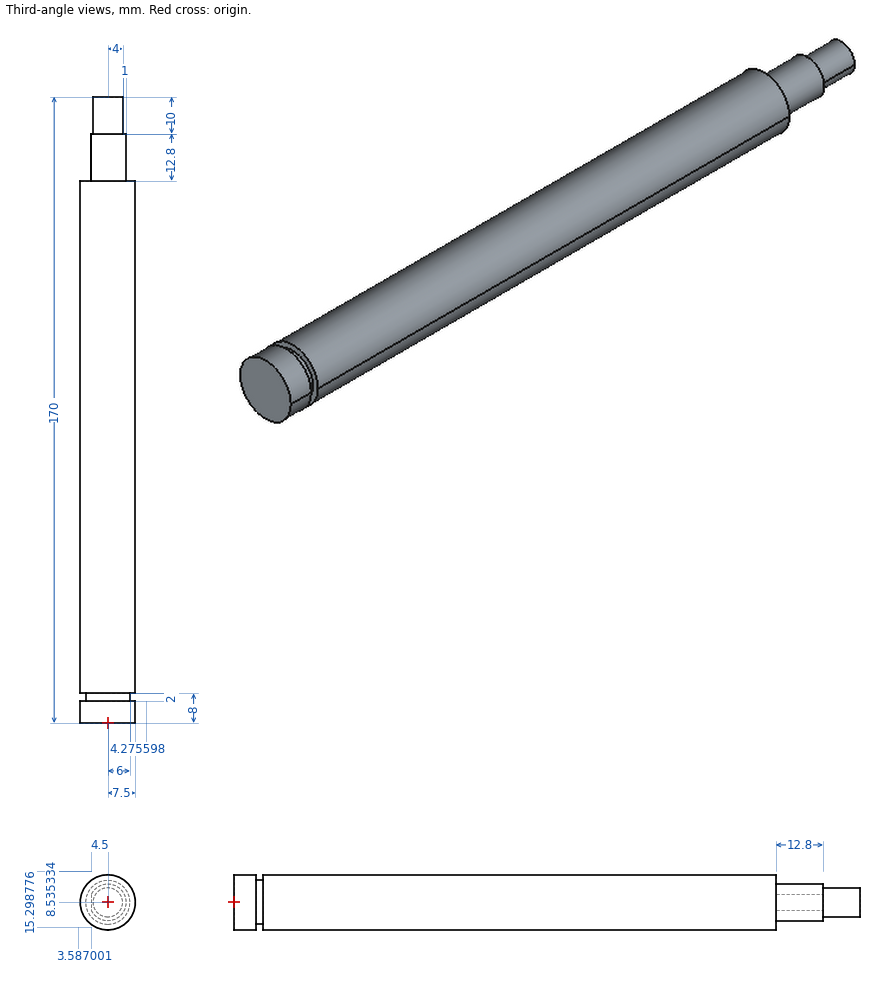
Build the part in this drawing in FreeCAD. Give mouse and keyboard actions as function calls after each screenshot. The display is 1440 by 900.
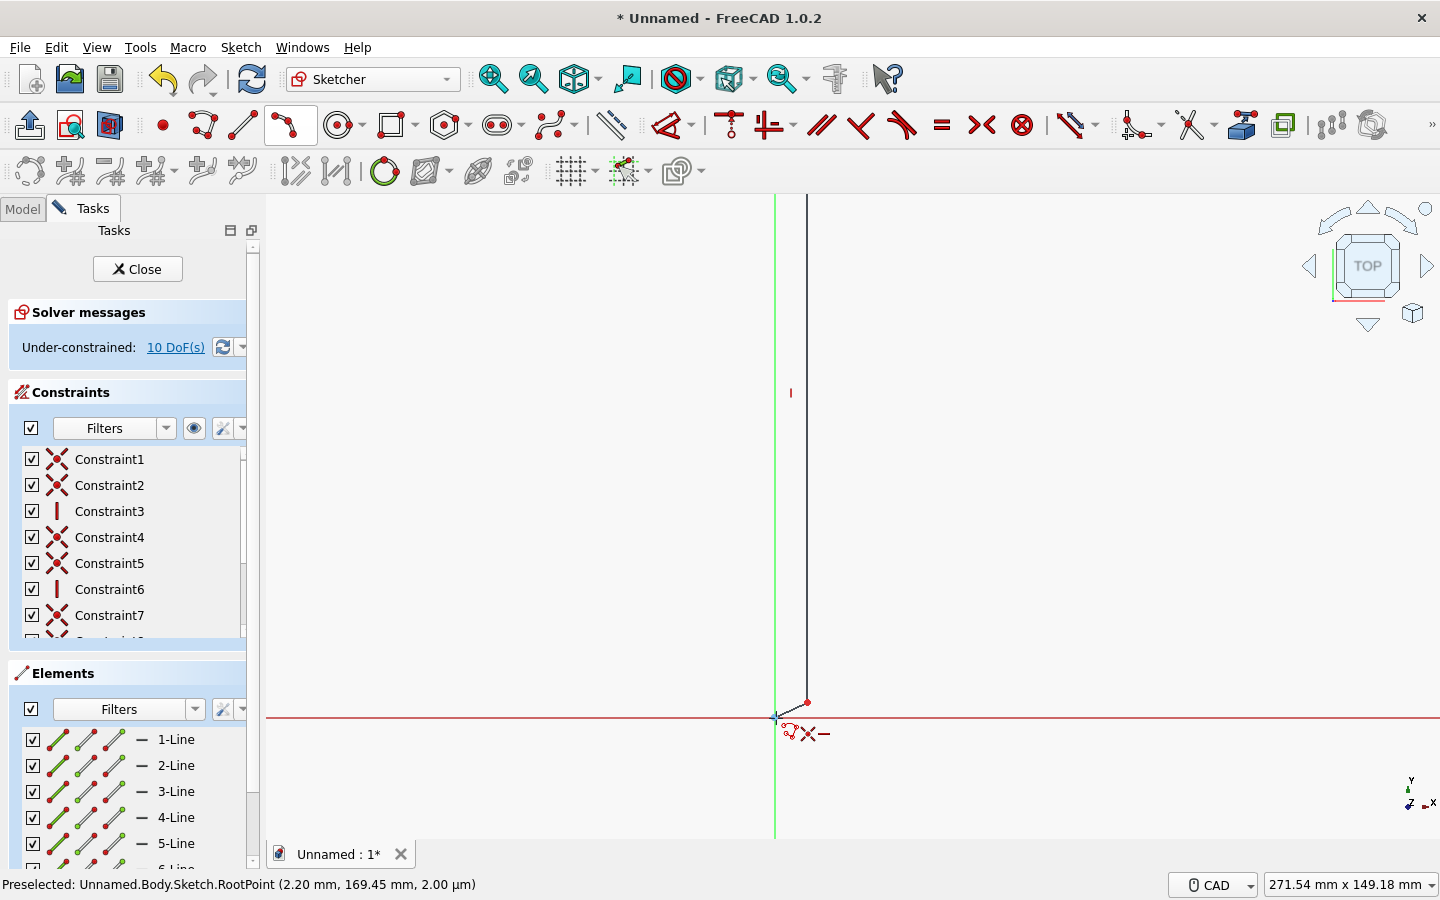
click(775, 718)
key(Escape)
key(Escape)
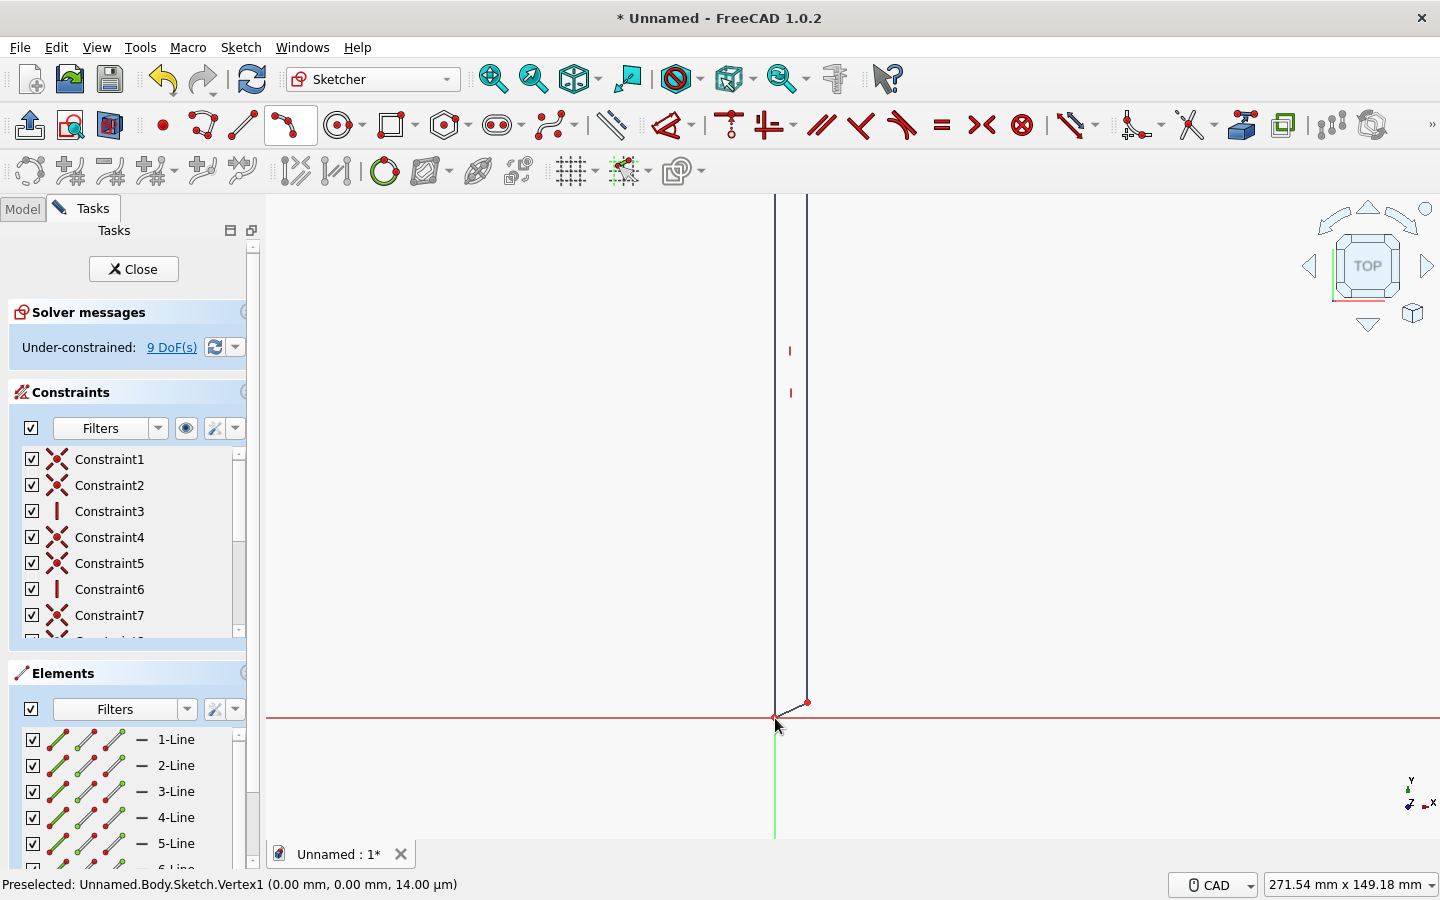
scroll(798, 707, up, 2)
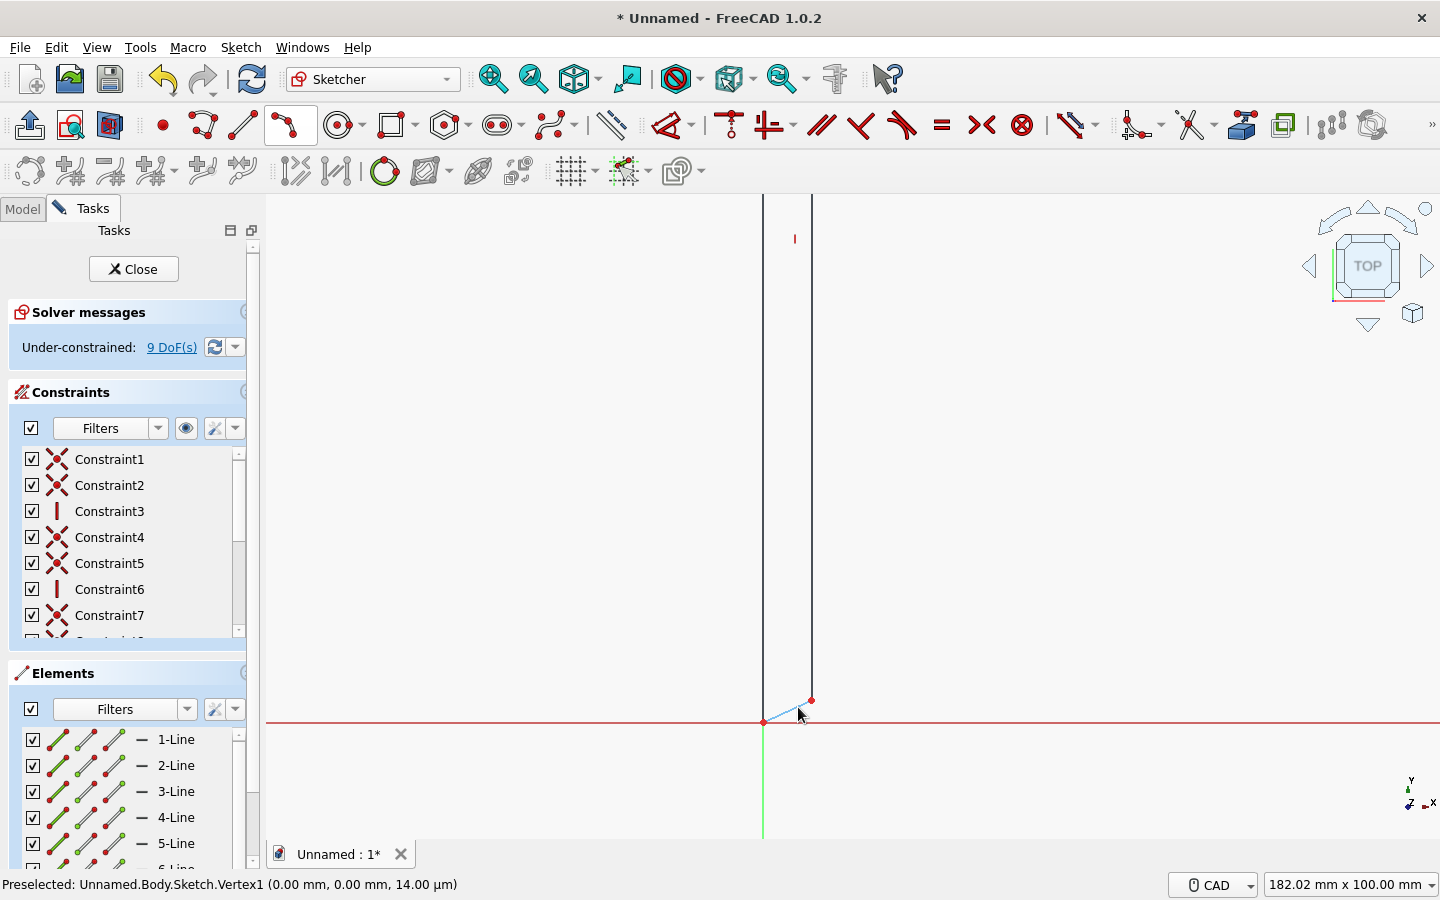
click(797, 707)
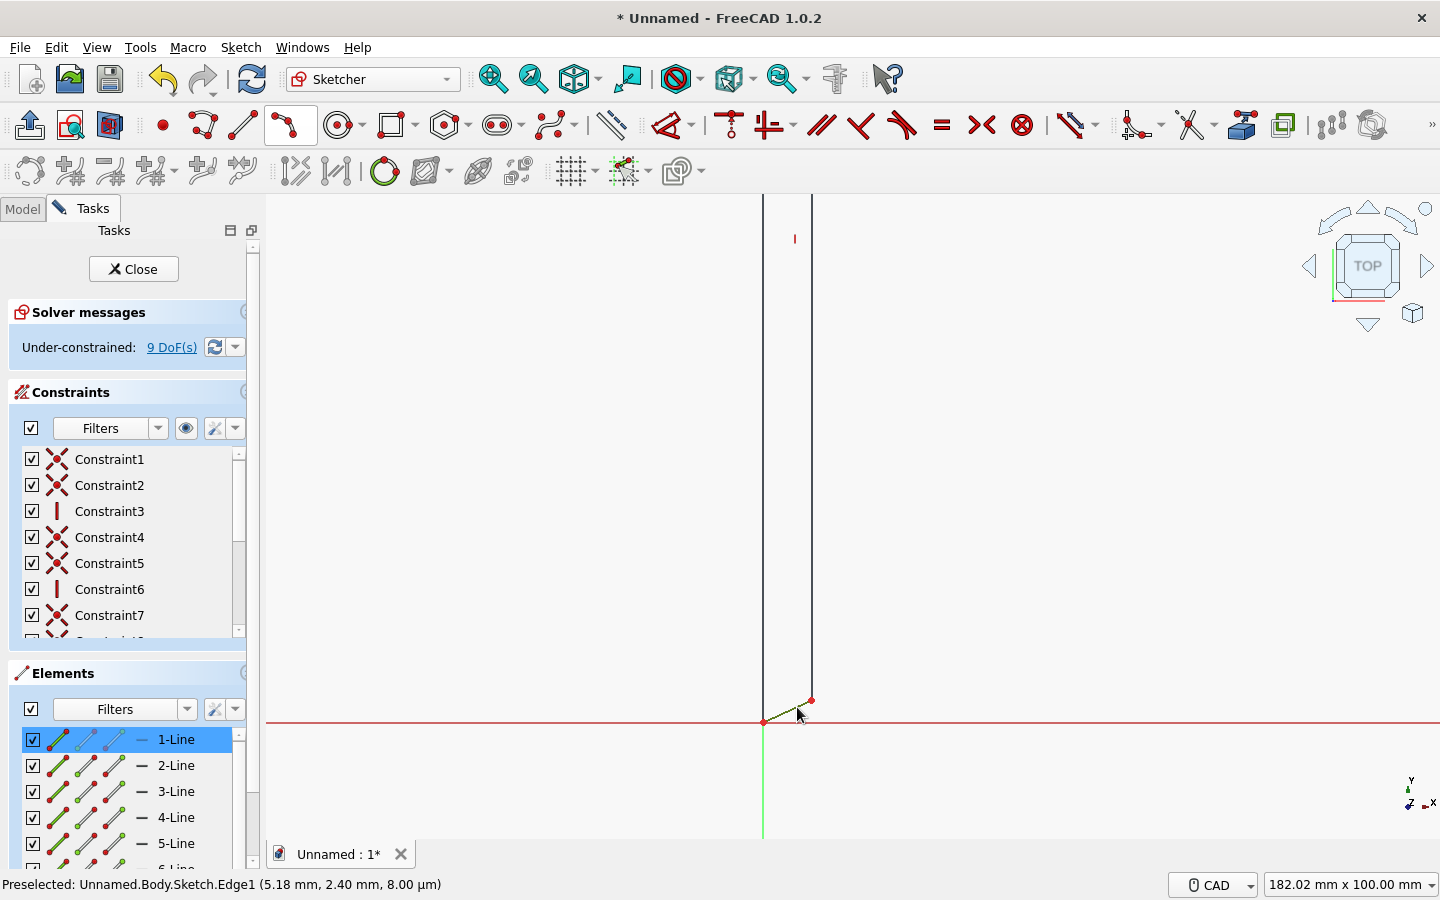
click(796, 126)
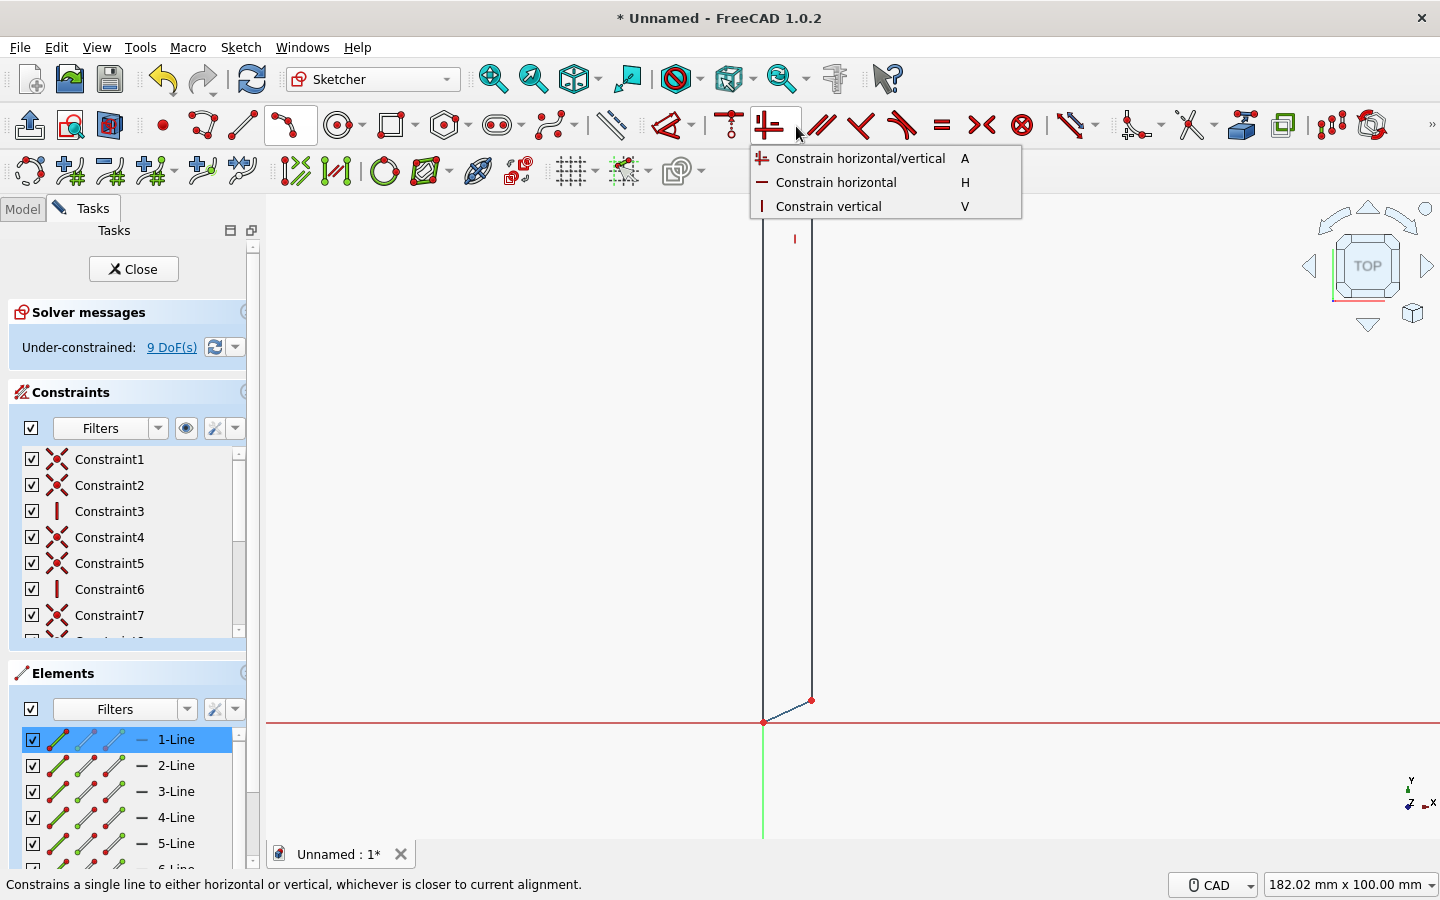
click(886, 182)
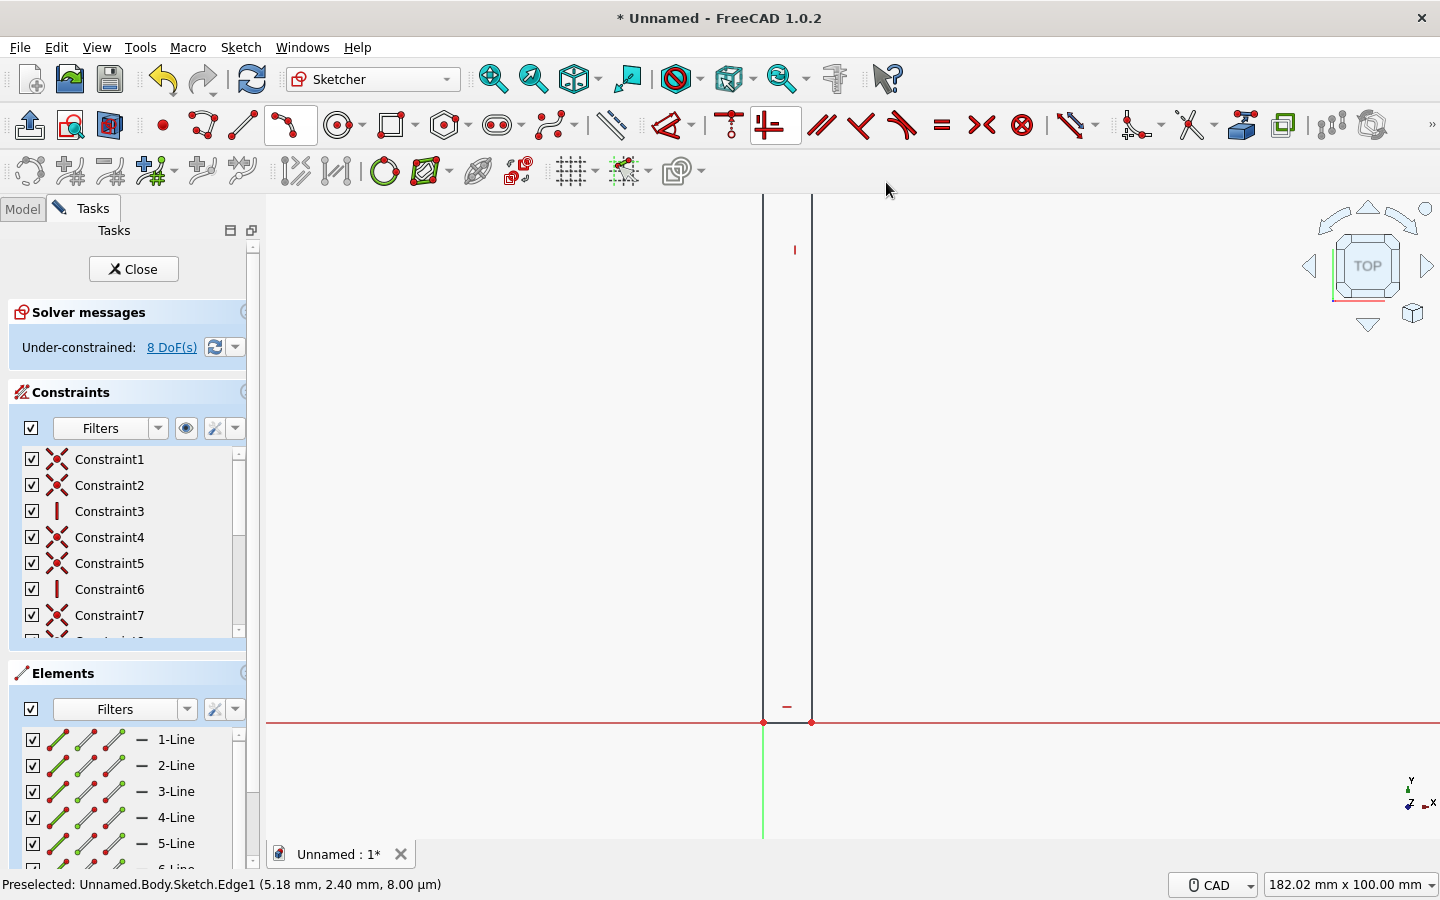
scroll(783, 716, down, 5)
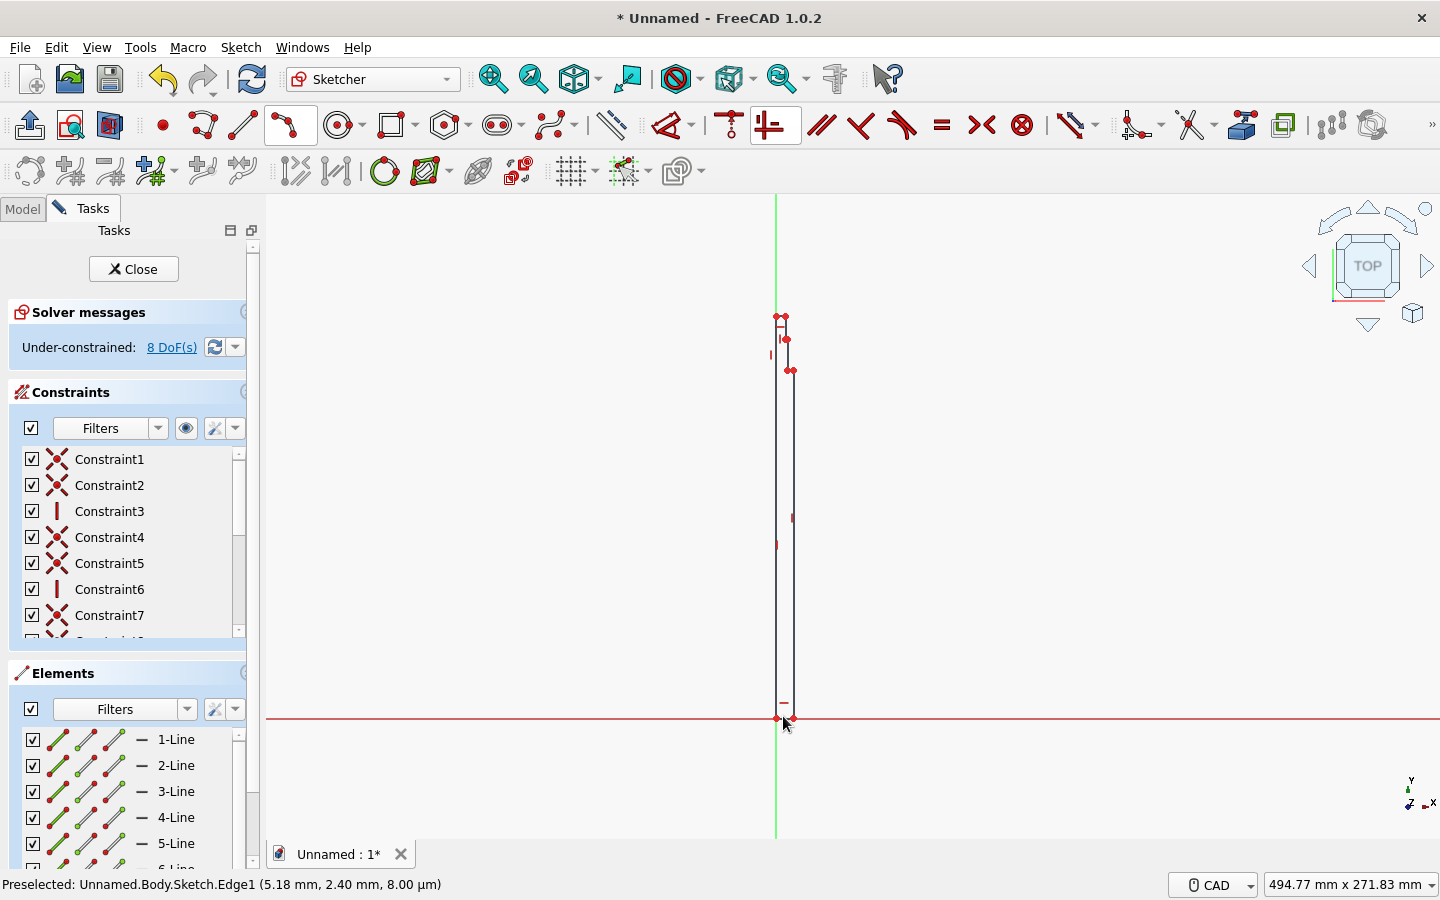
scroll(791, 370, up, 8)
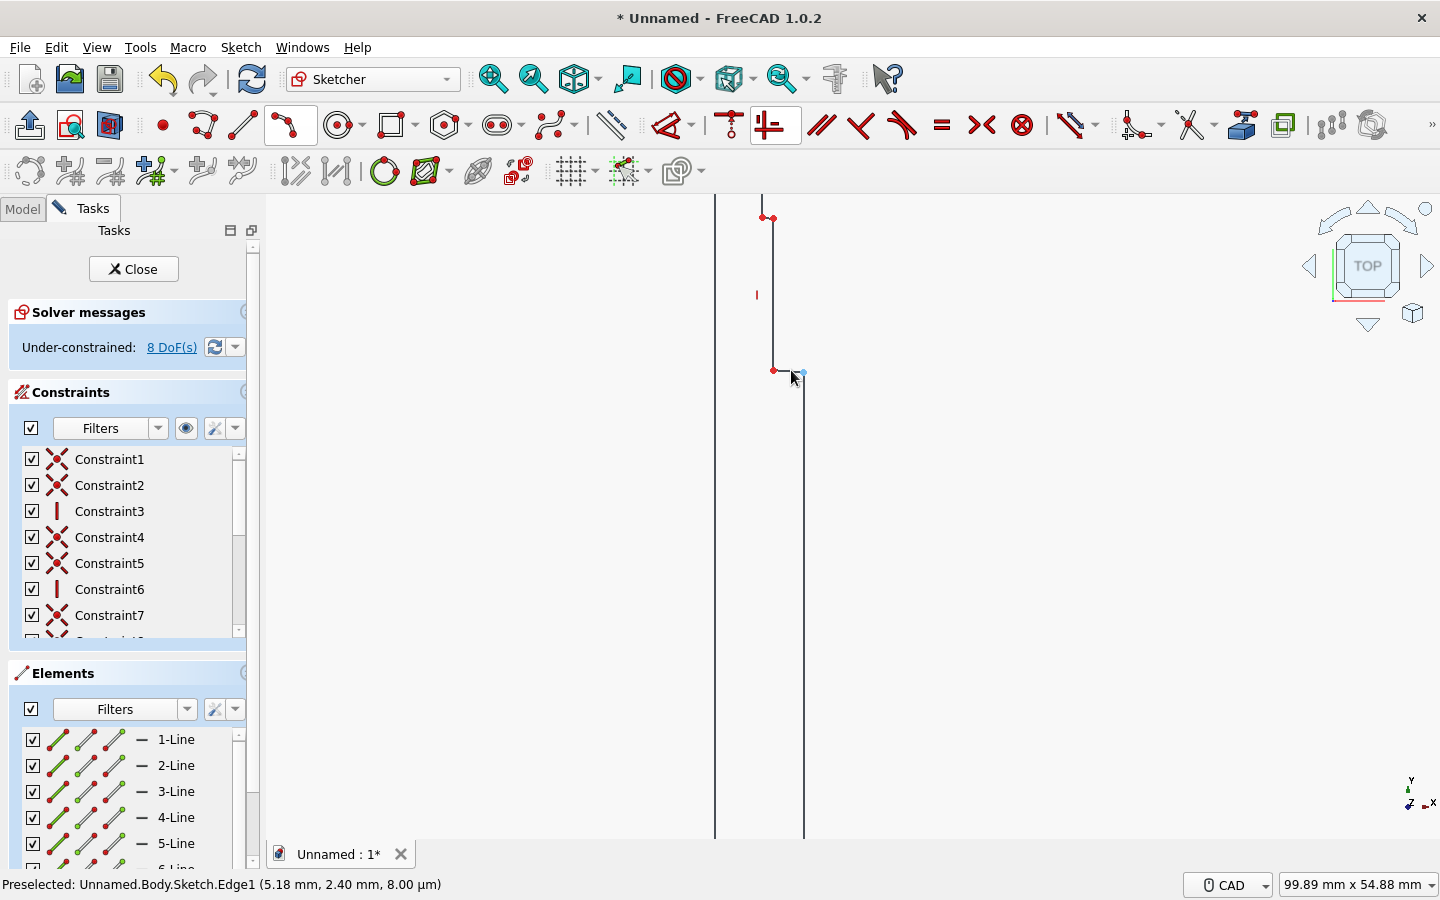
click(788, 371)